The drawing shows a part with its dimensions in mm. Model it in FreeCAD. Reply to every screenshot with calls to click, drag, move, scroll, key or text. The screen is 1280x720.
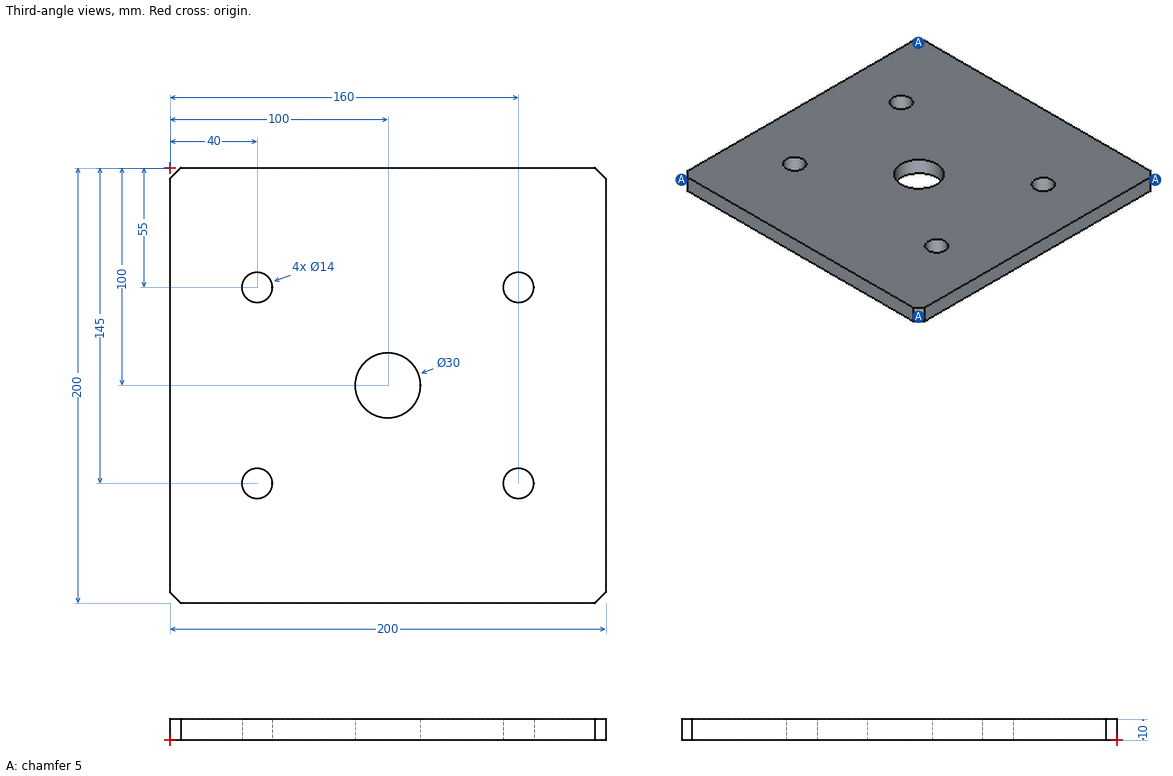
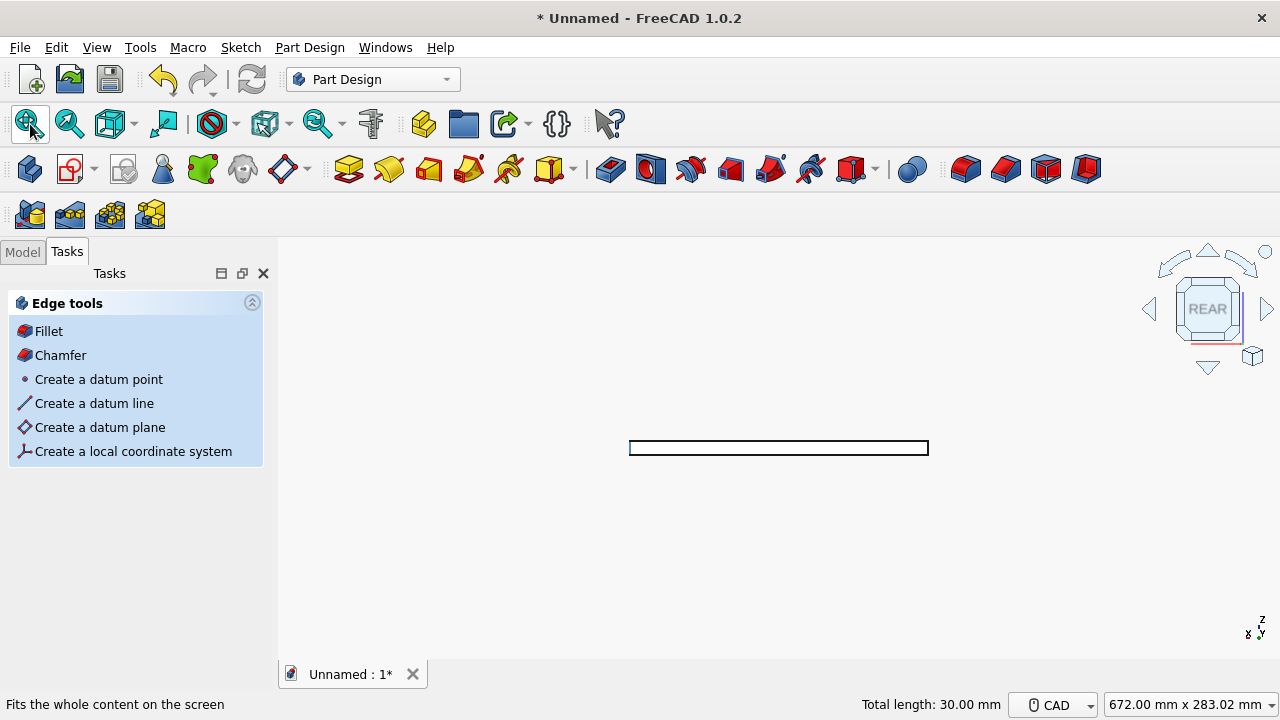
click(30, 124)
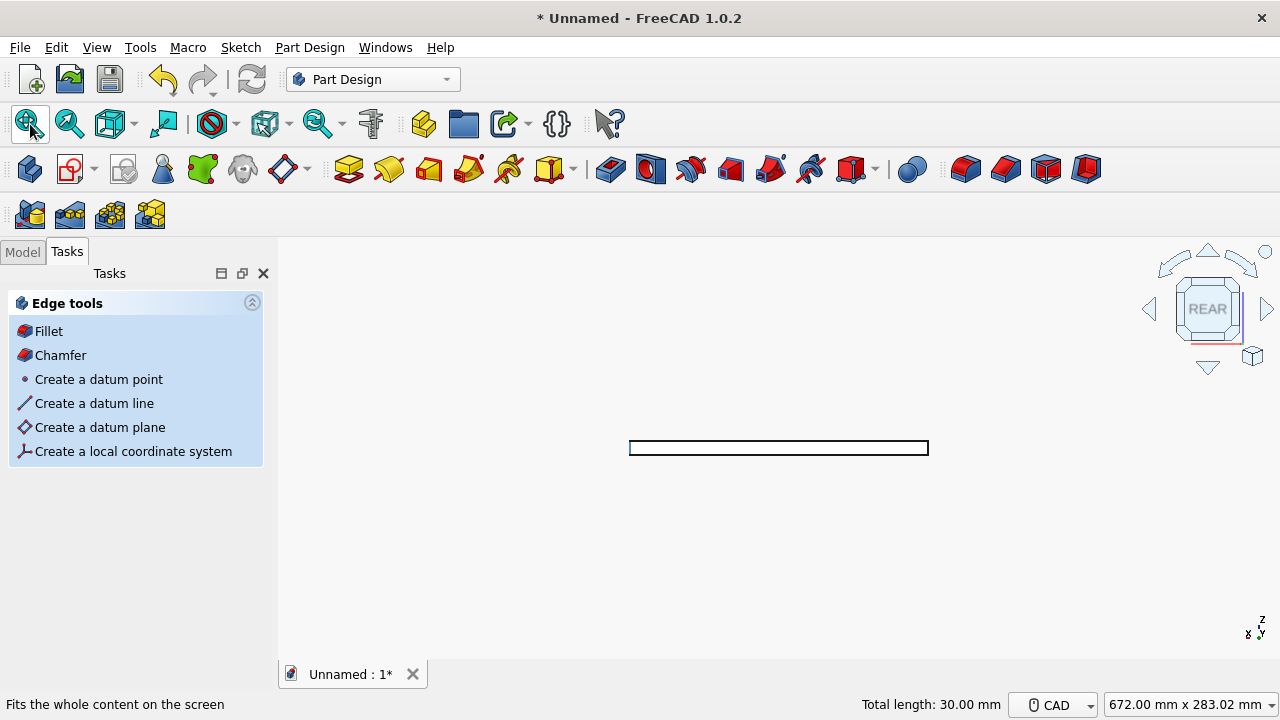
click(928, 447, ctrl)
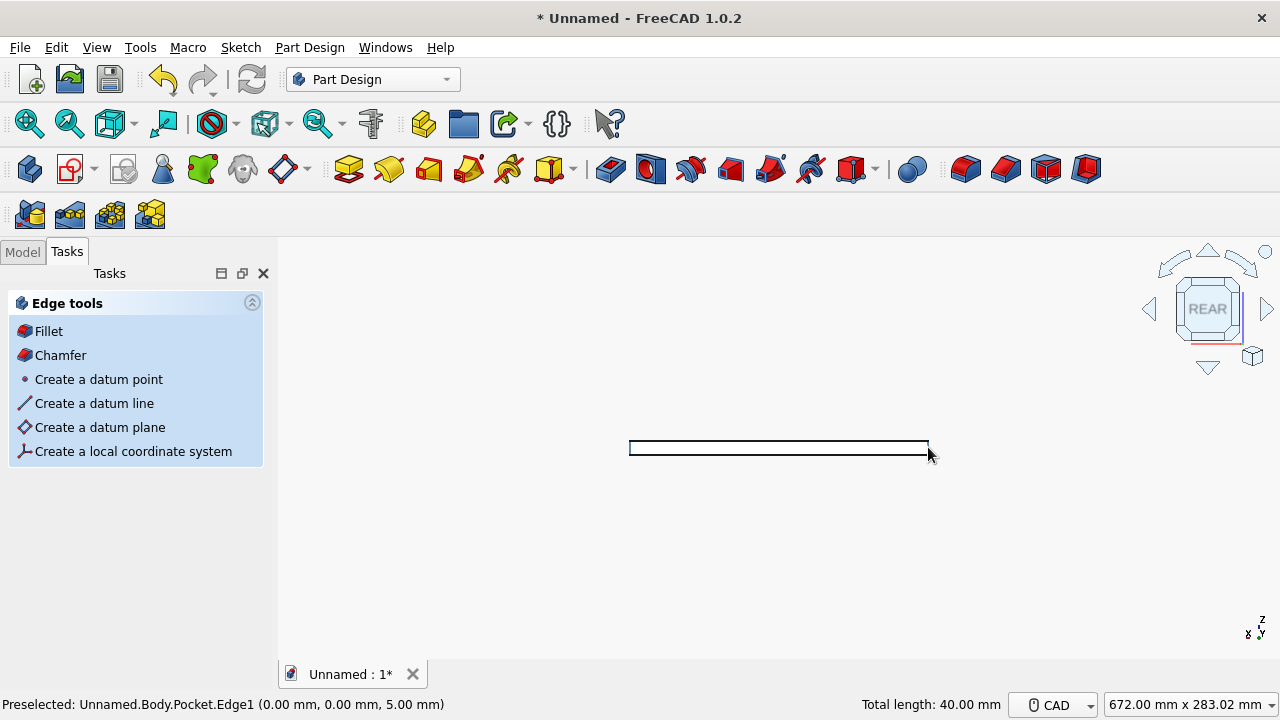
click(1006, 170)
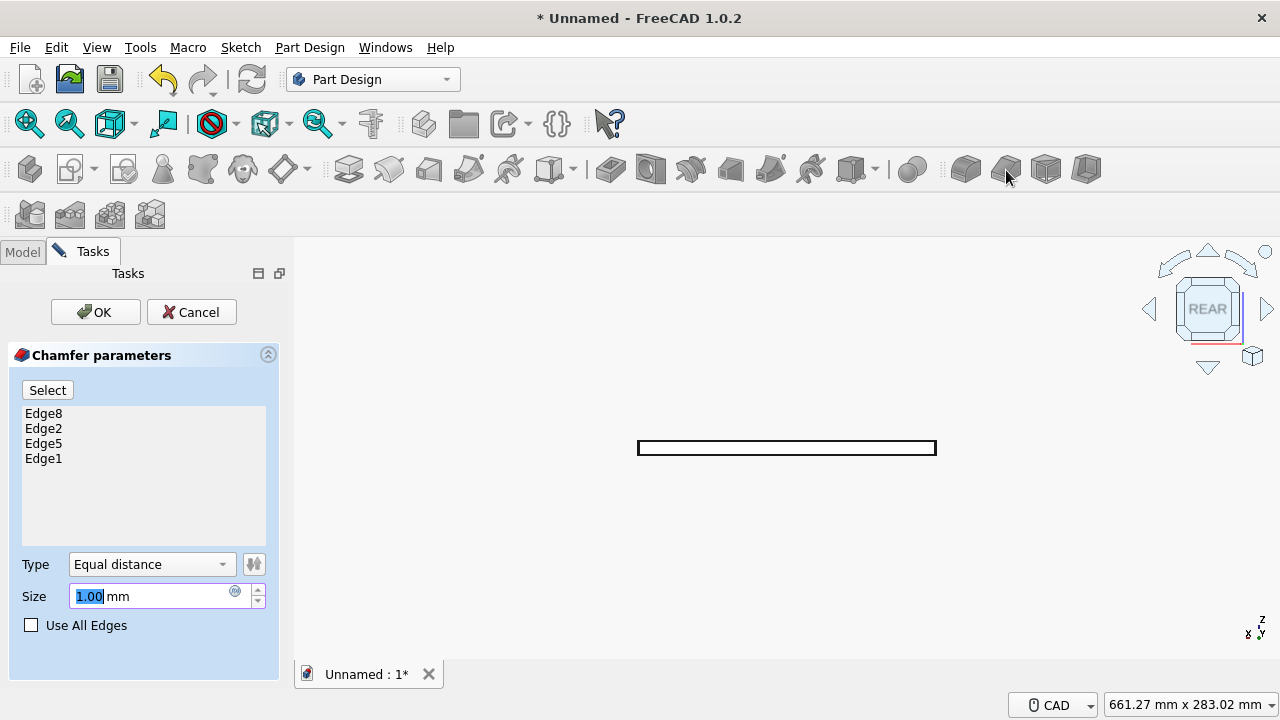
text(5)
key(Tab)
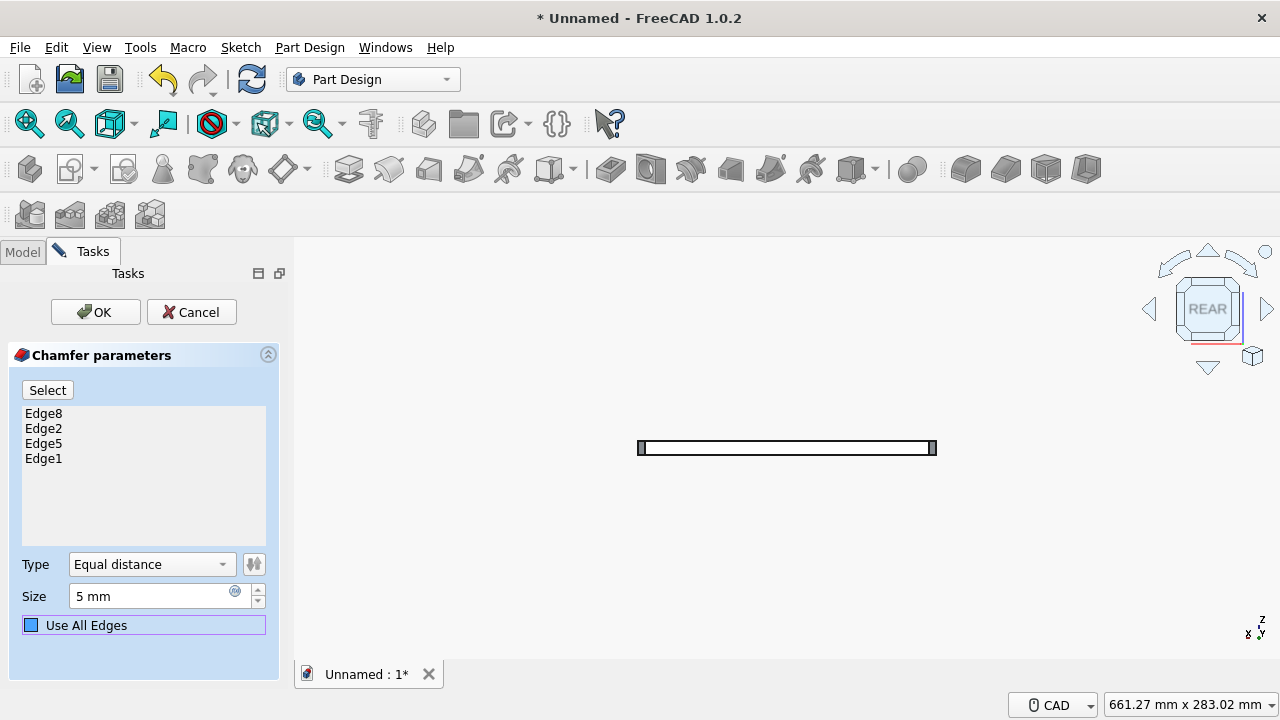
click(96, 312)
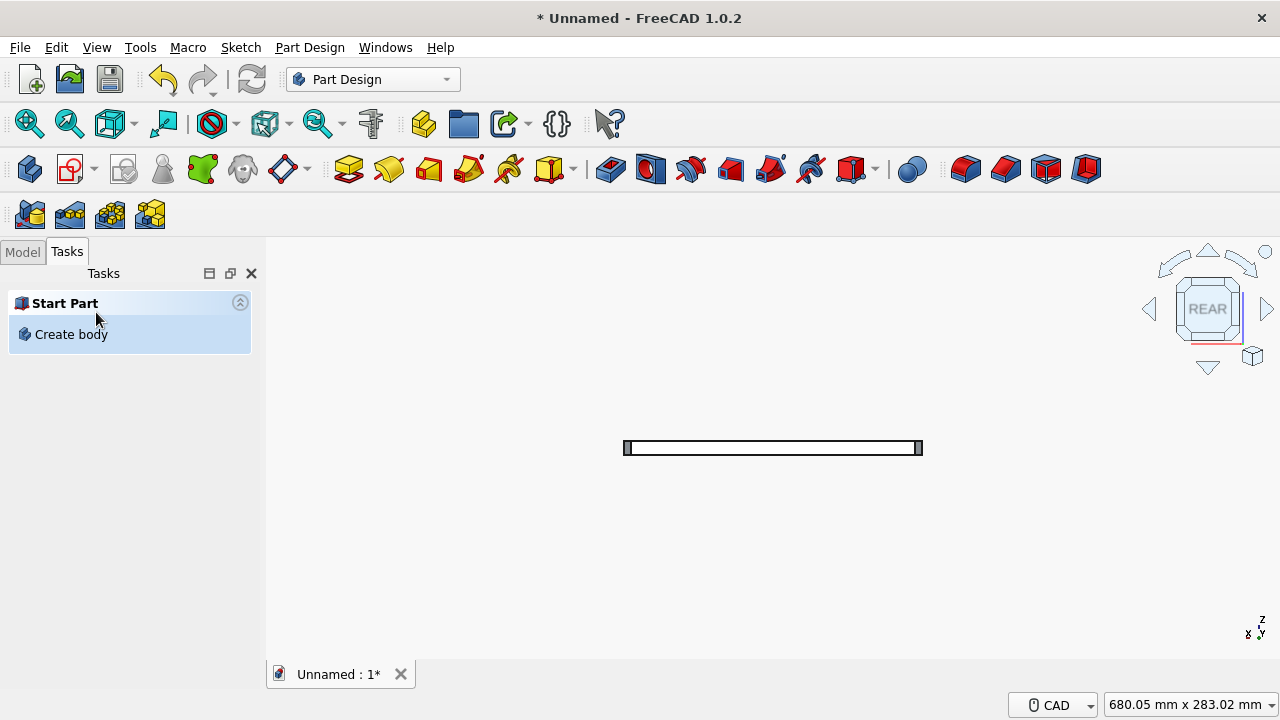
key(0)